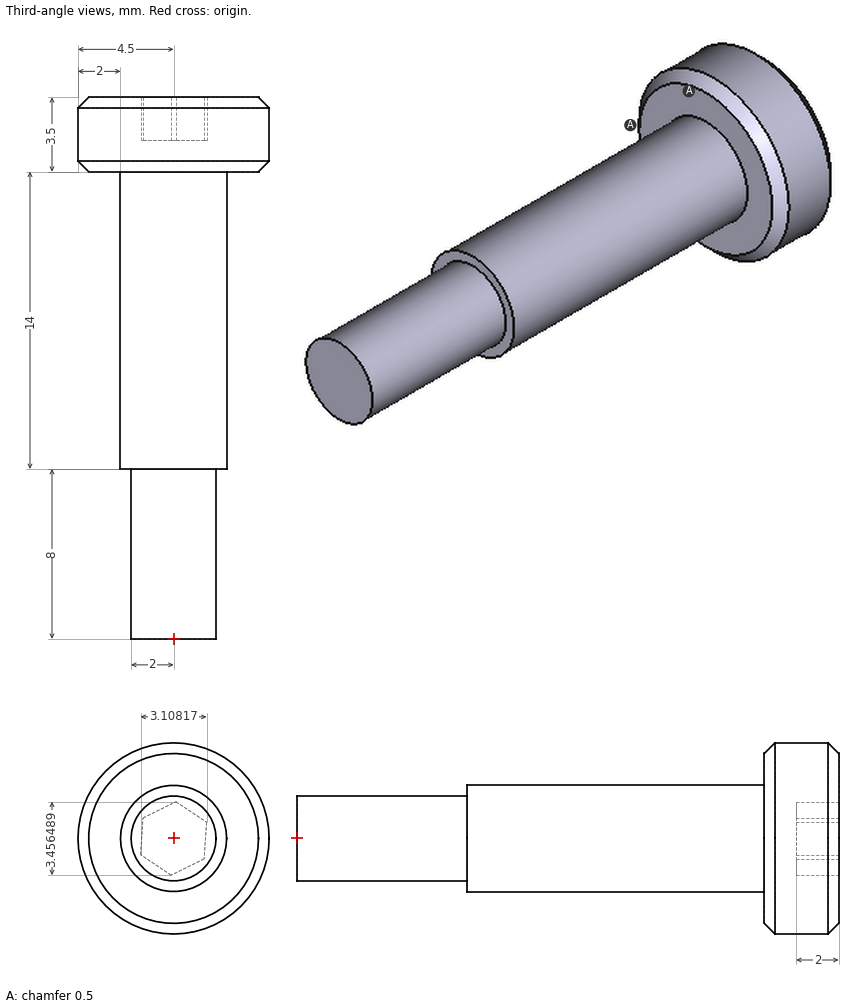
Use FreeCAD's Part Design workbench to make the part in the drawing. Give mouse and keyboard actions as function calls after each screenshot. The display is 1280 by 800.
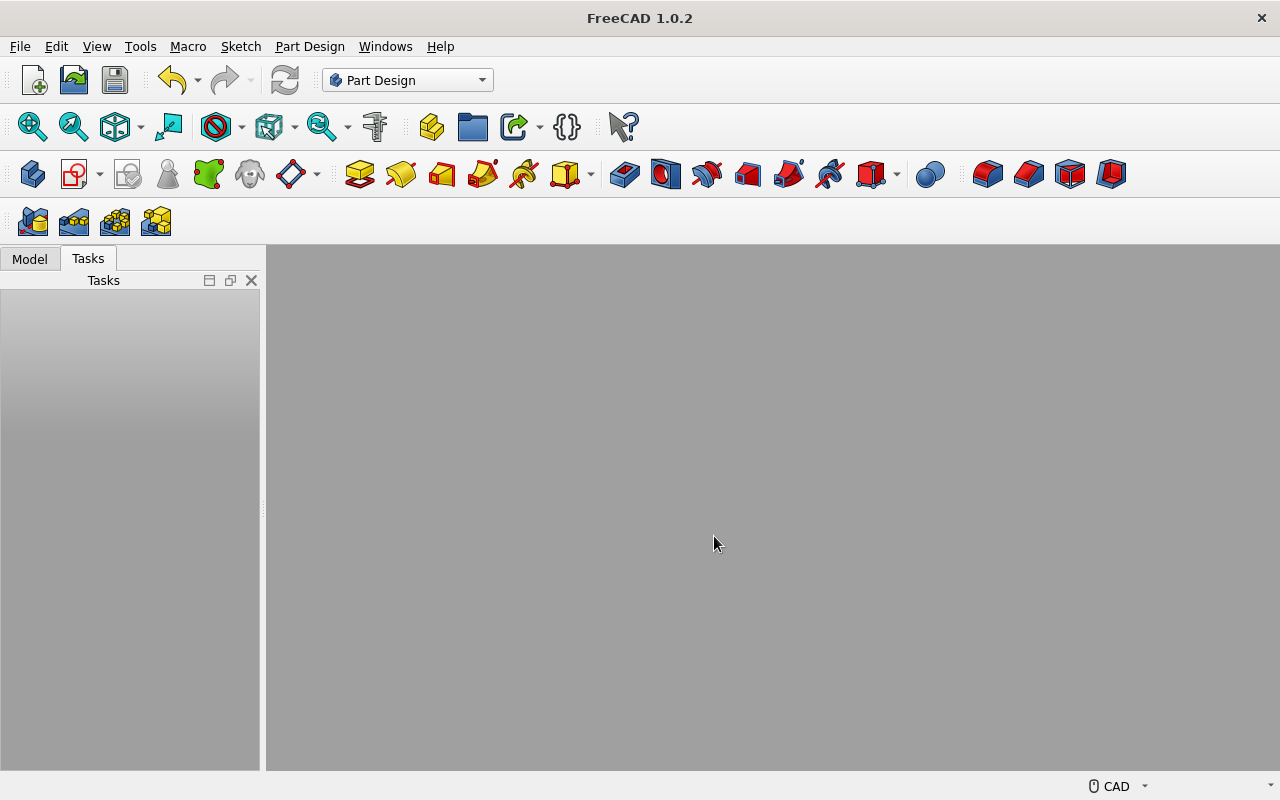
click(33, 80)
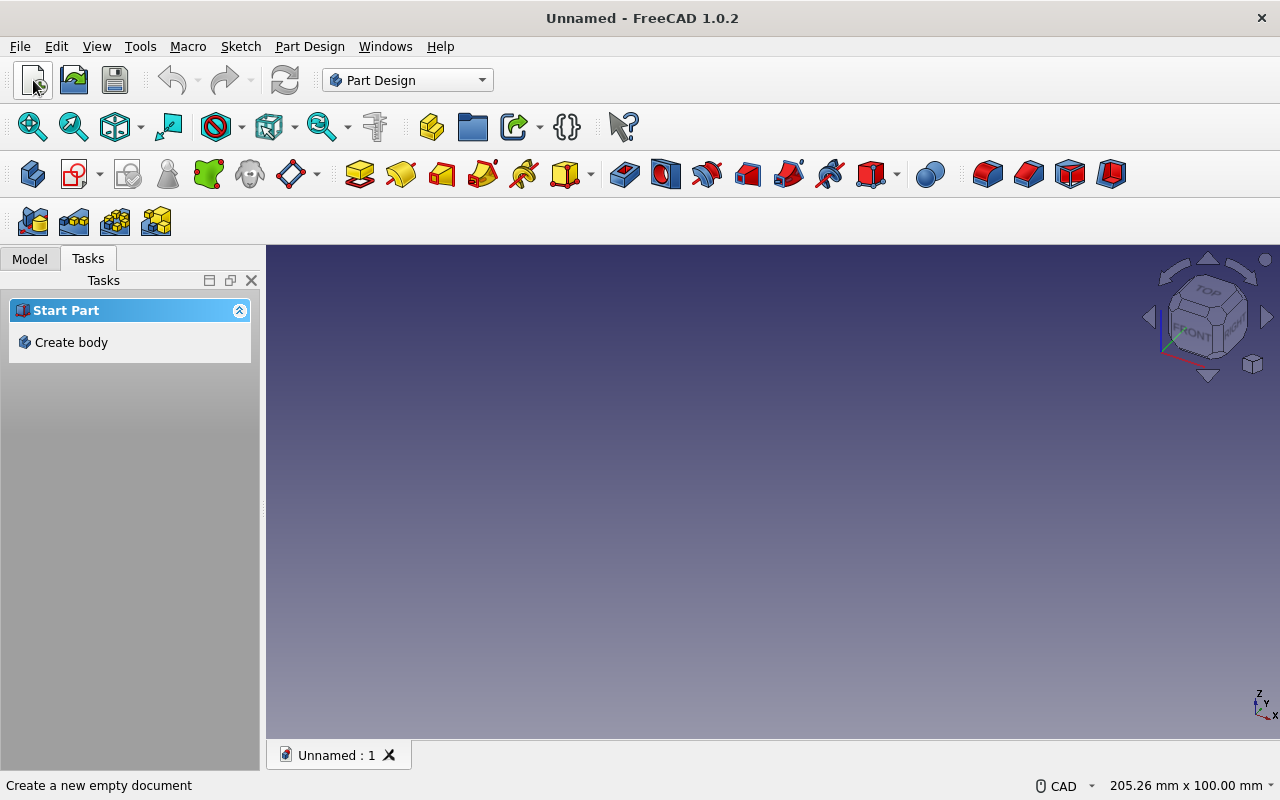
click(74, 174)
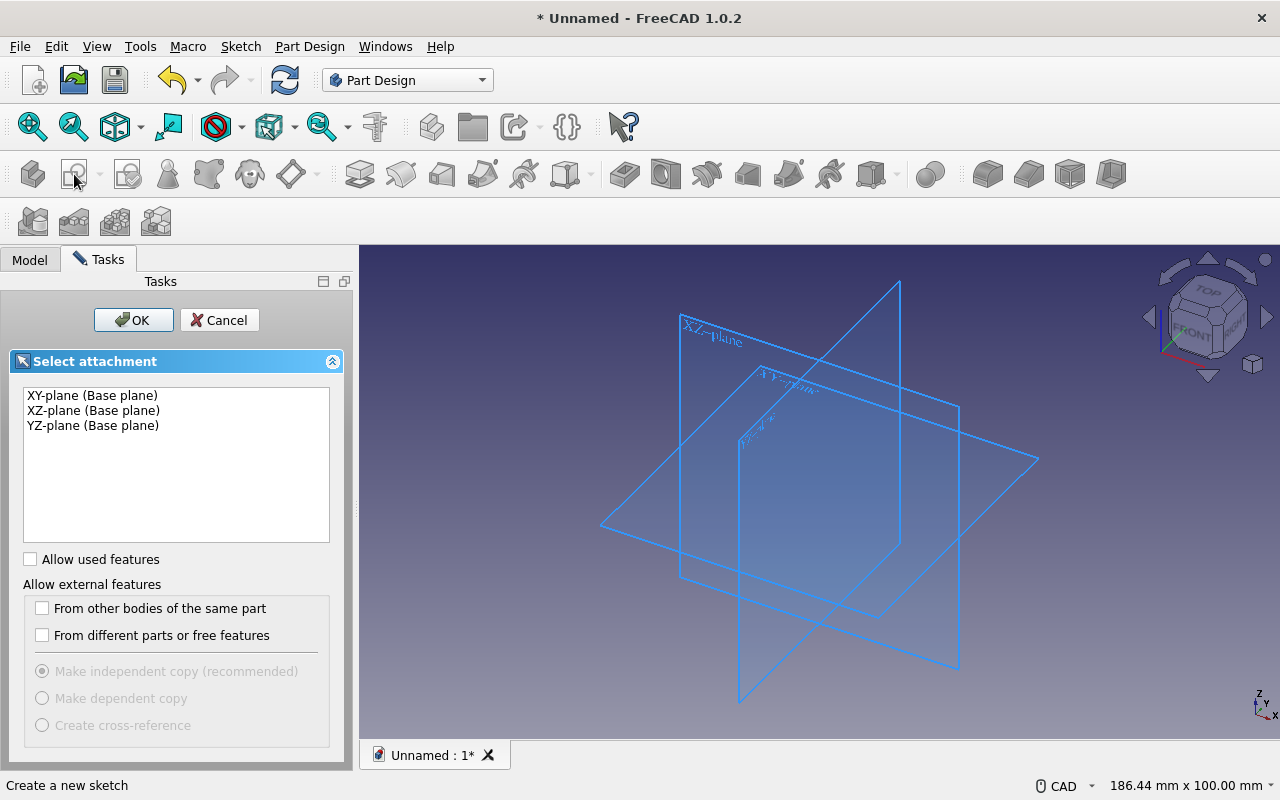
click(84, 396)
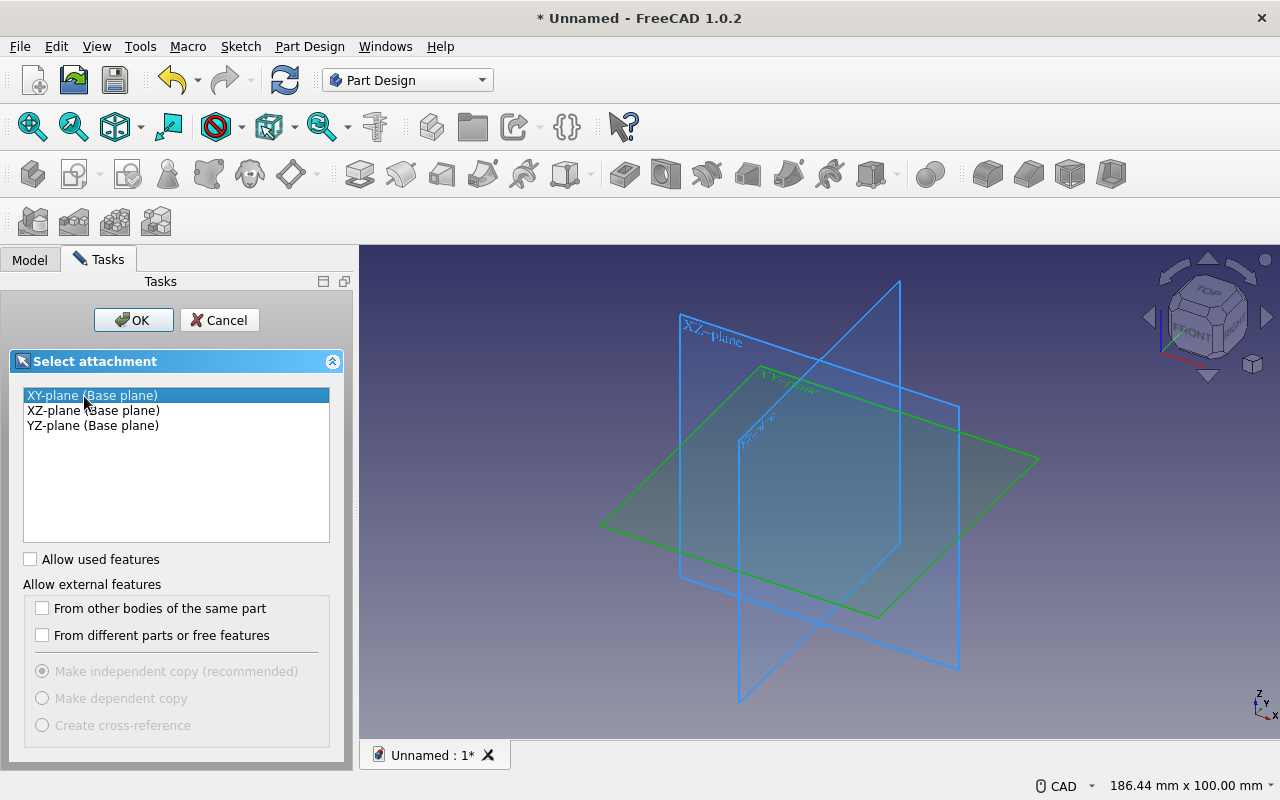
click(134, 320)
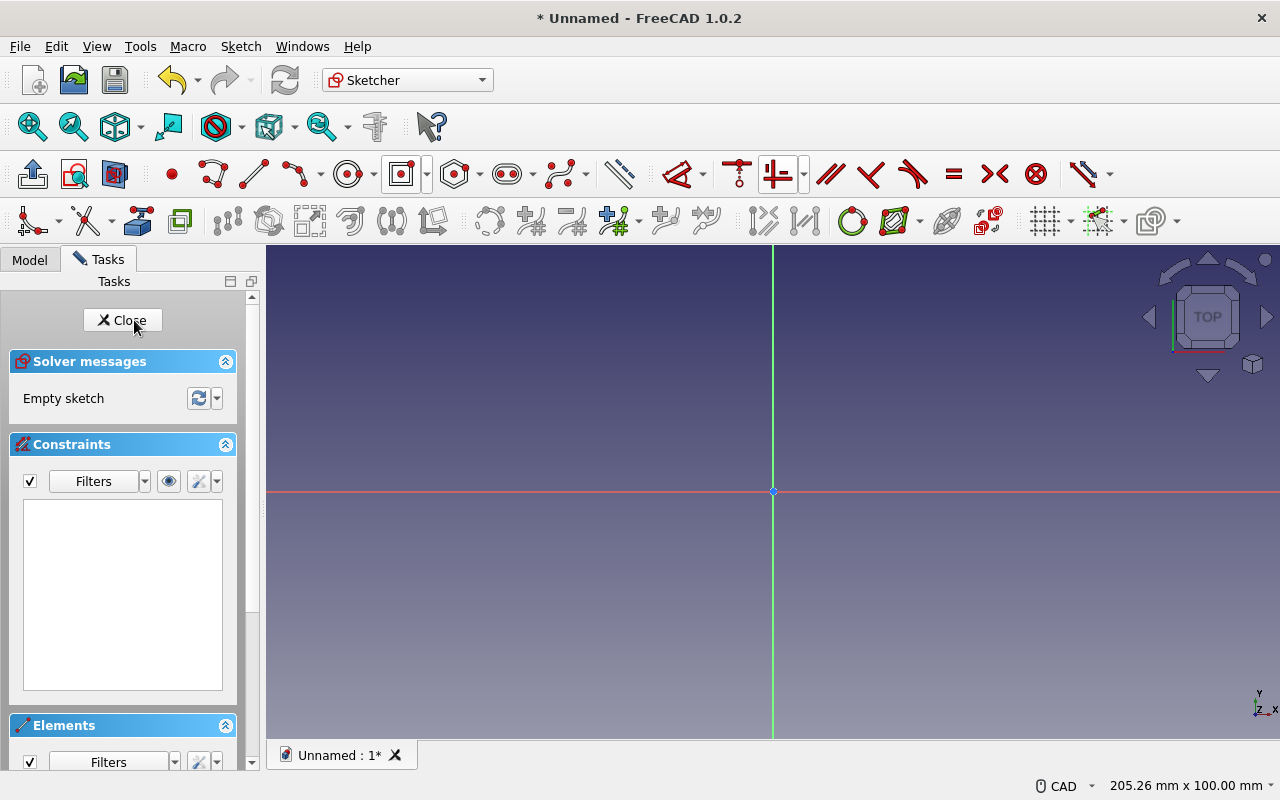
scroll(809, 378, up, 4)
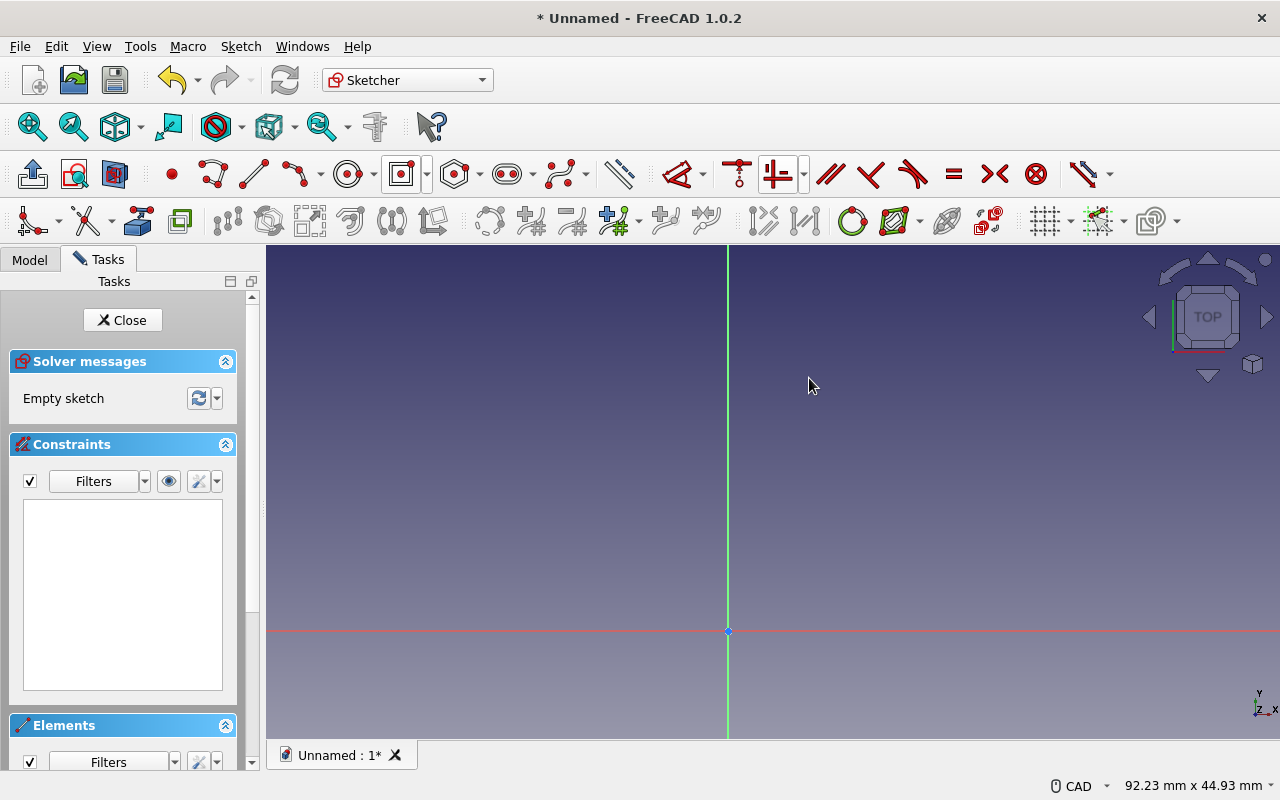
click(213, 174)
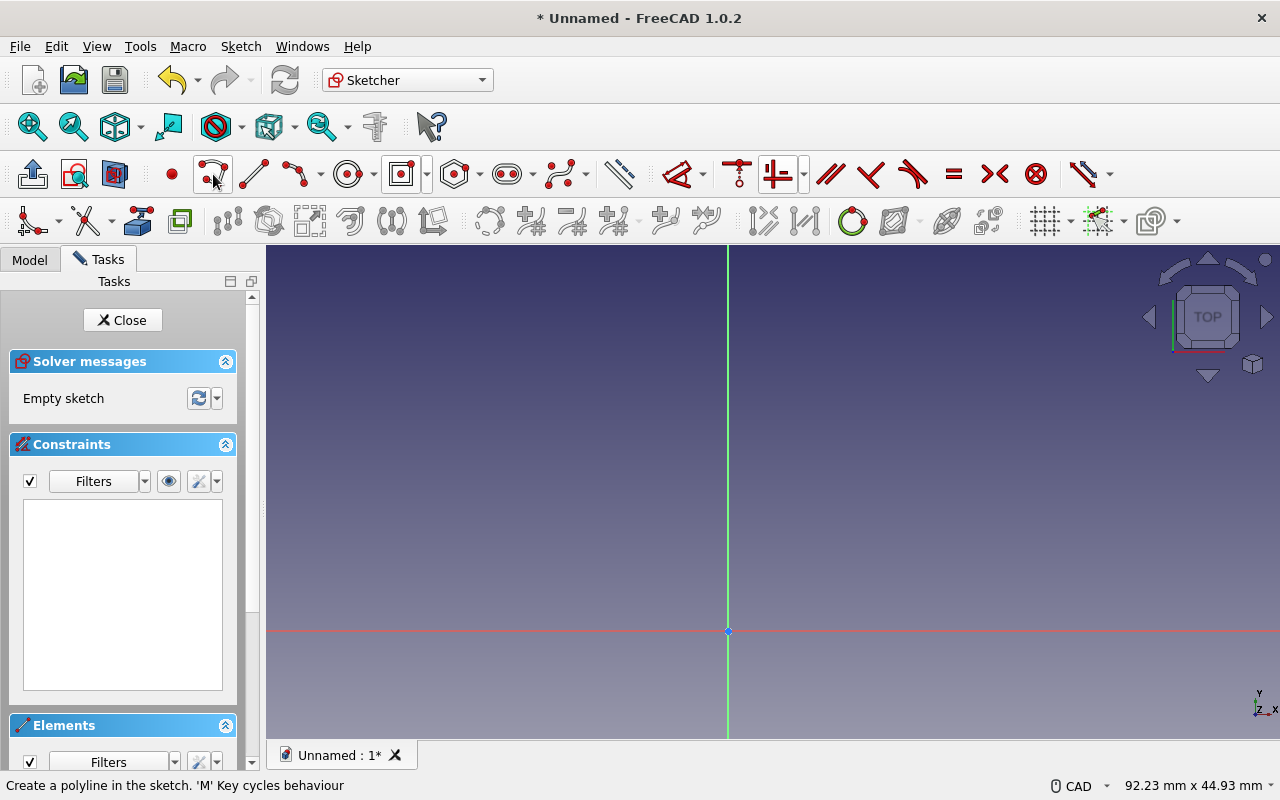
click(728, 631)
click(719, 351)
click(679, 351)
click(679, 390)
click(701, 390)
click(701, 543)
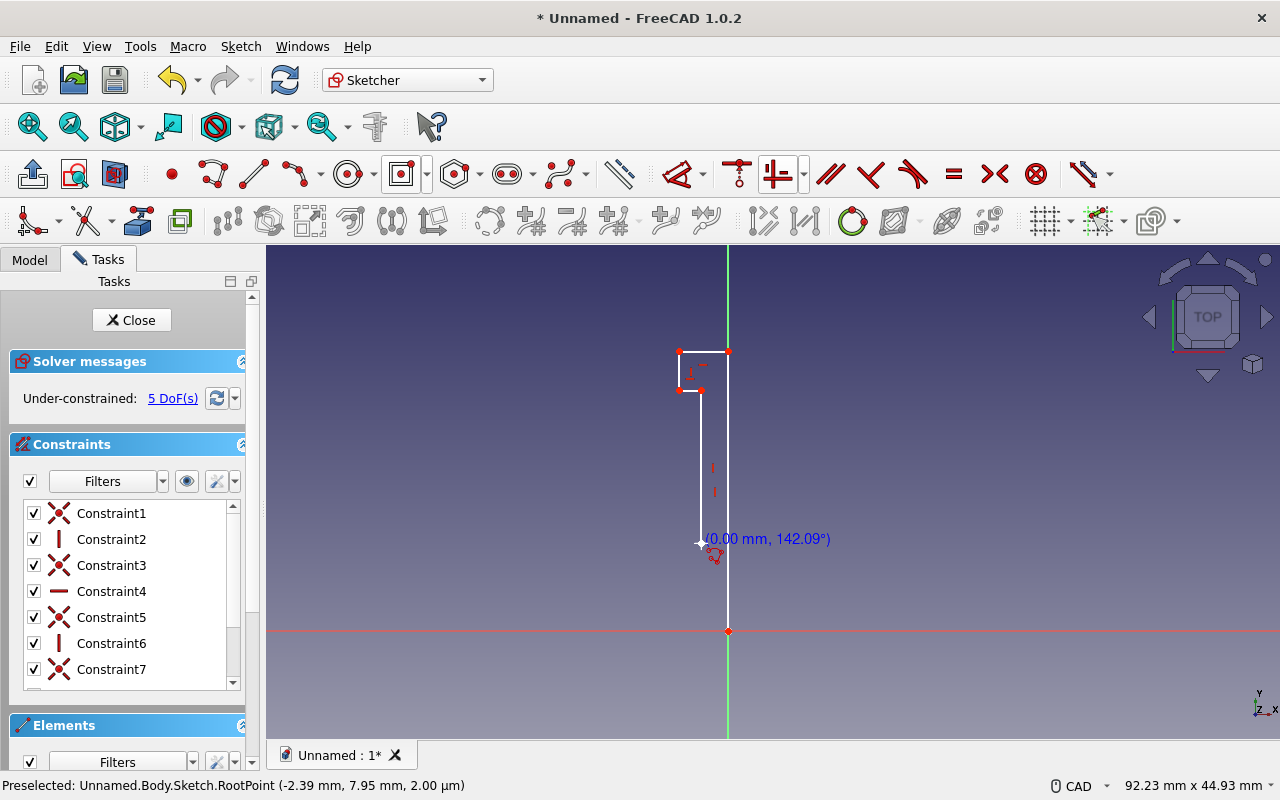
scroll(706, 543, up, 6)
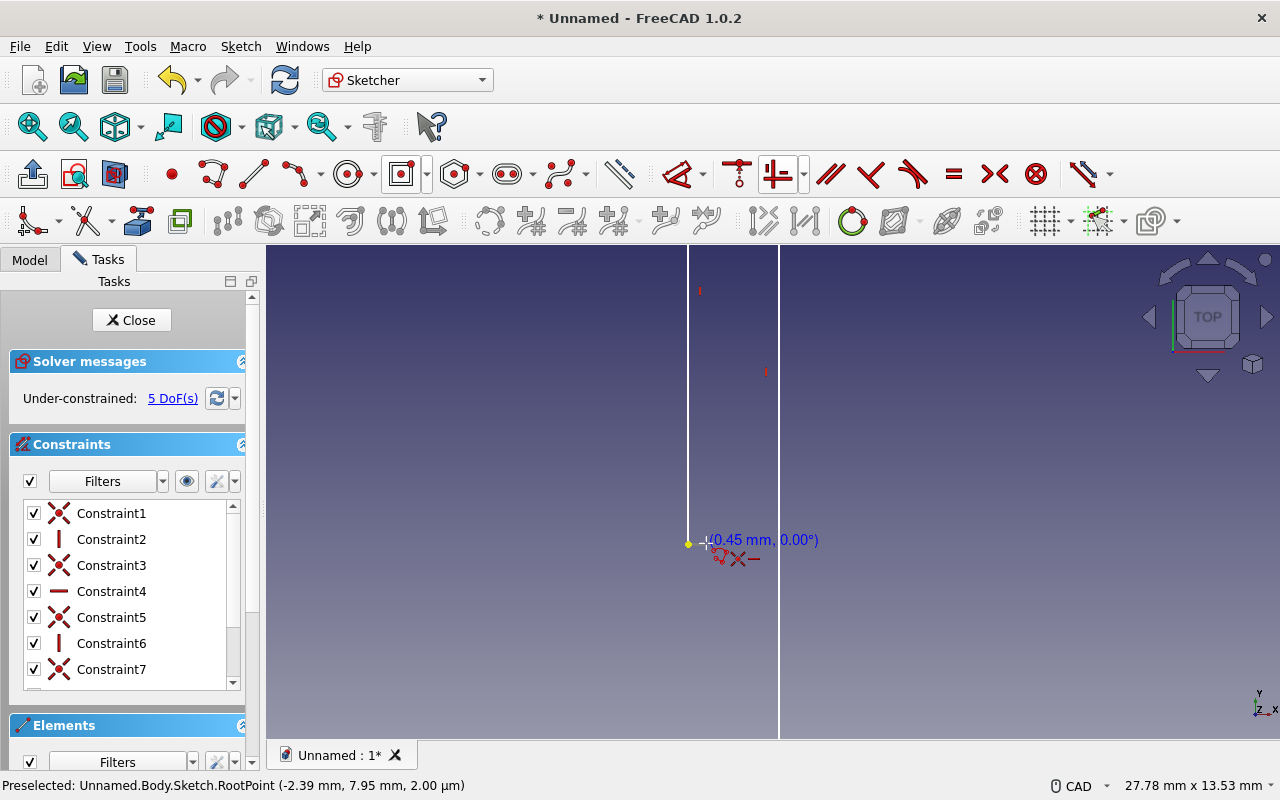
click(706, 542)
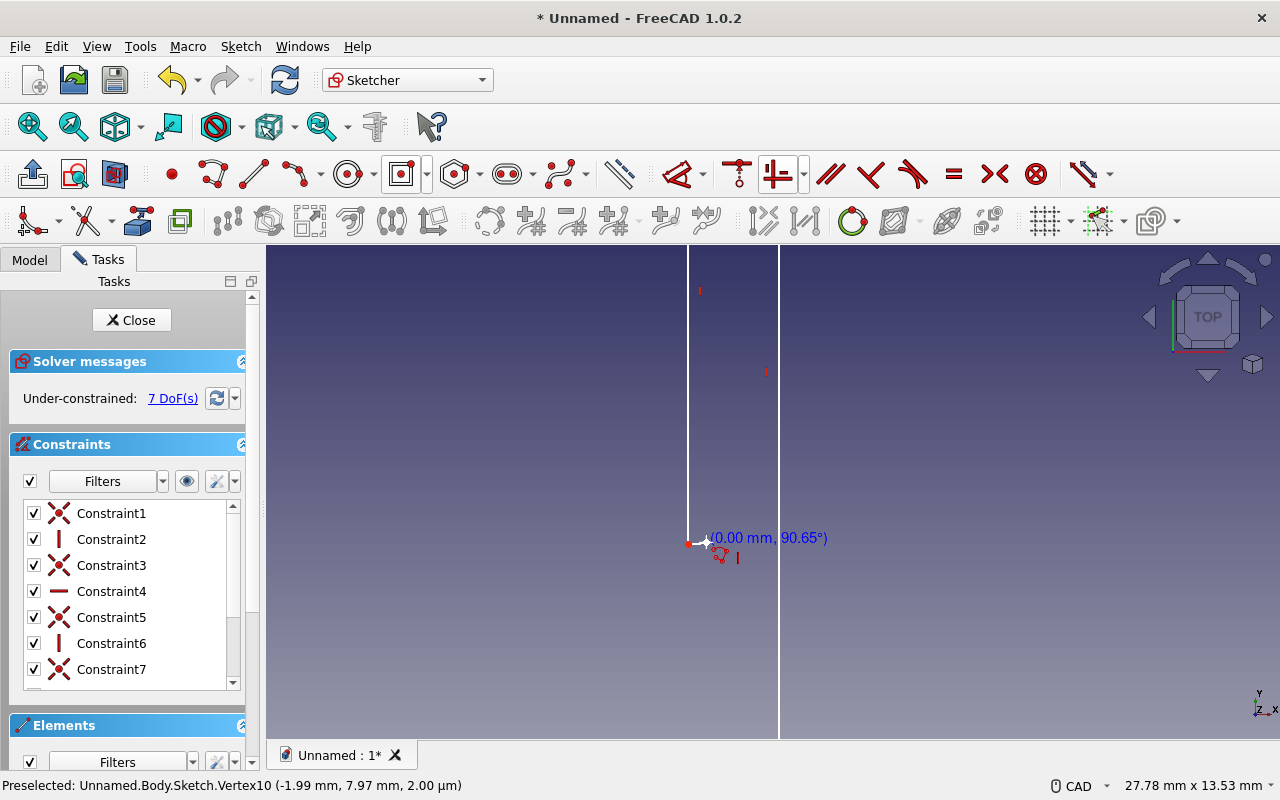
scroll(708, 545, down, 6)